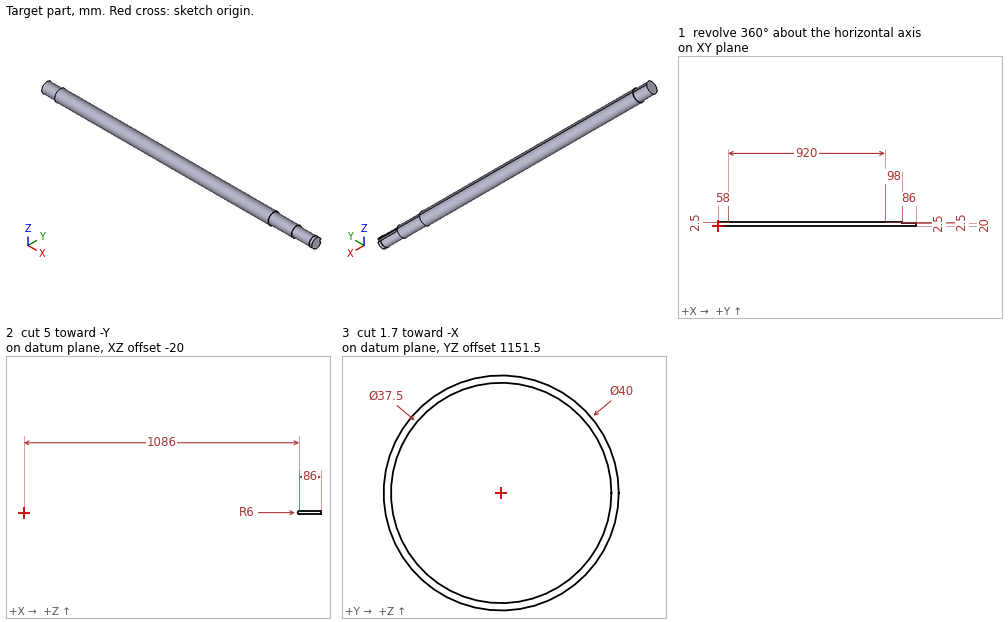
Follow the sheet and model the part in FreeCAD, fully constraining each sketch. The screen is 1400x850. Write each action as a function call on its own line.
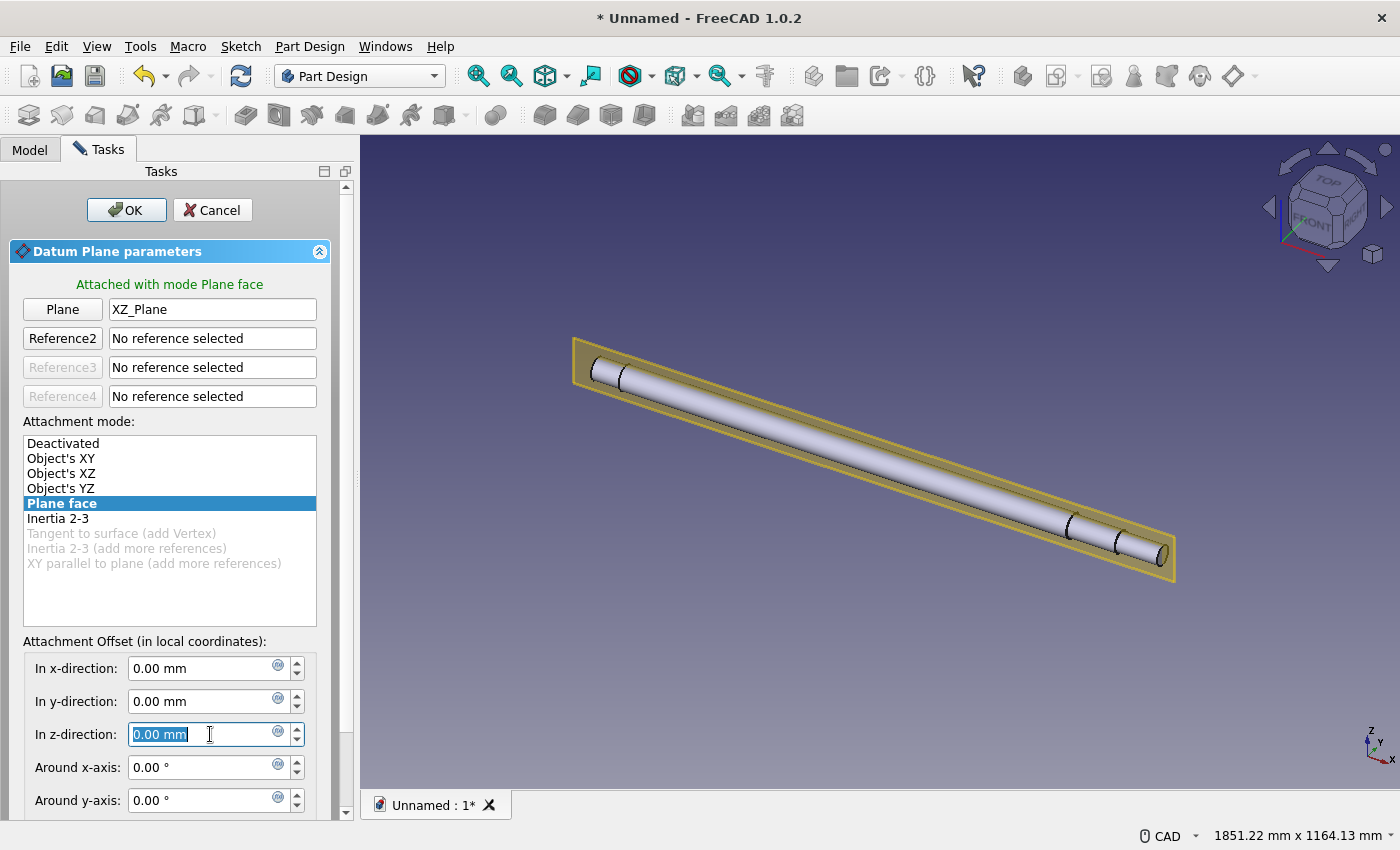
text(-20)
key(Tab)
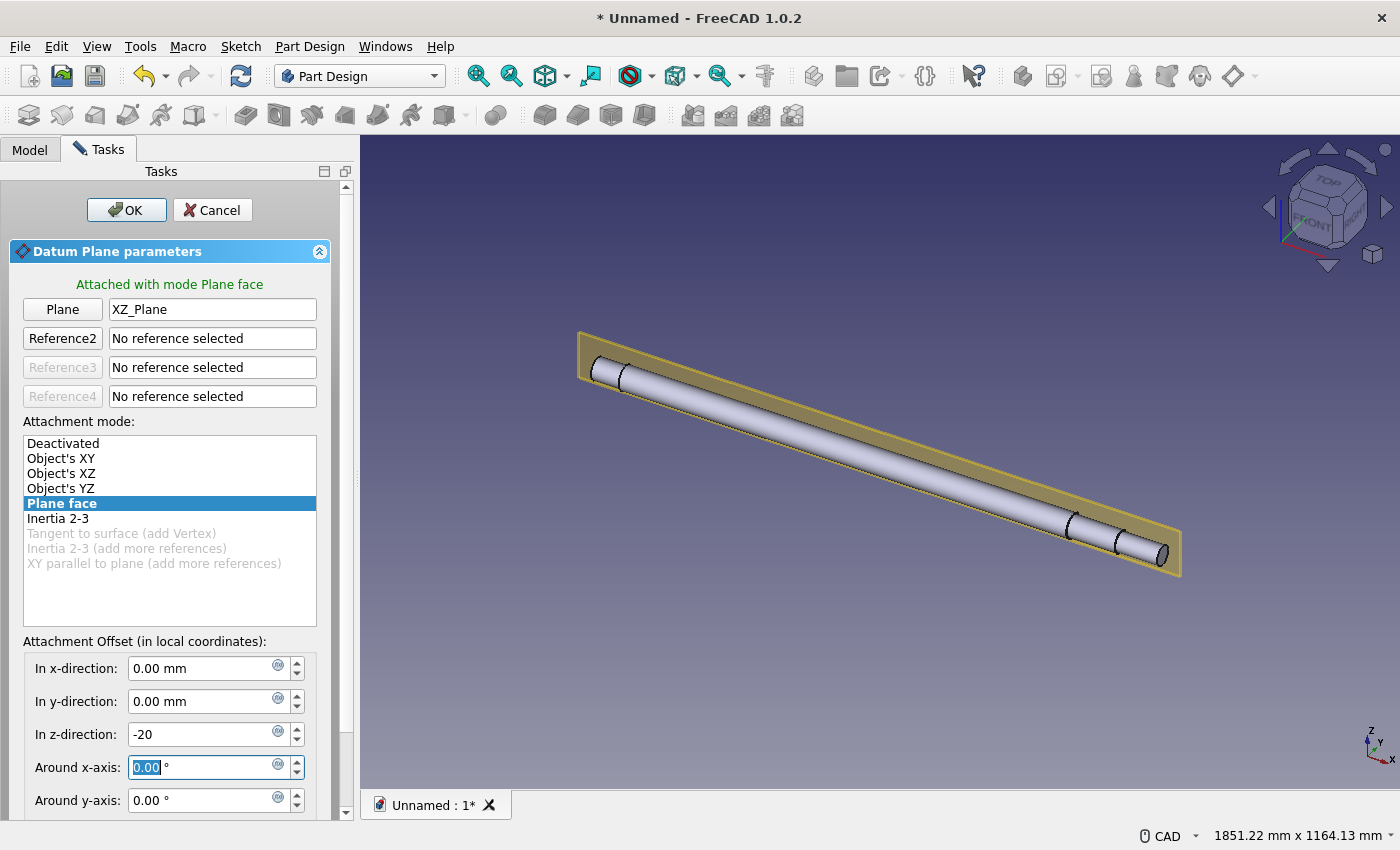
click(127, 210)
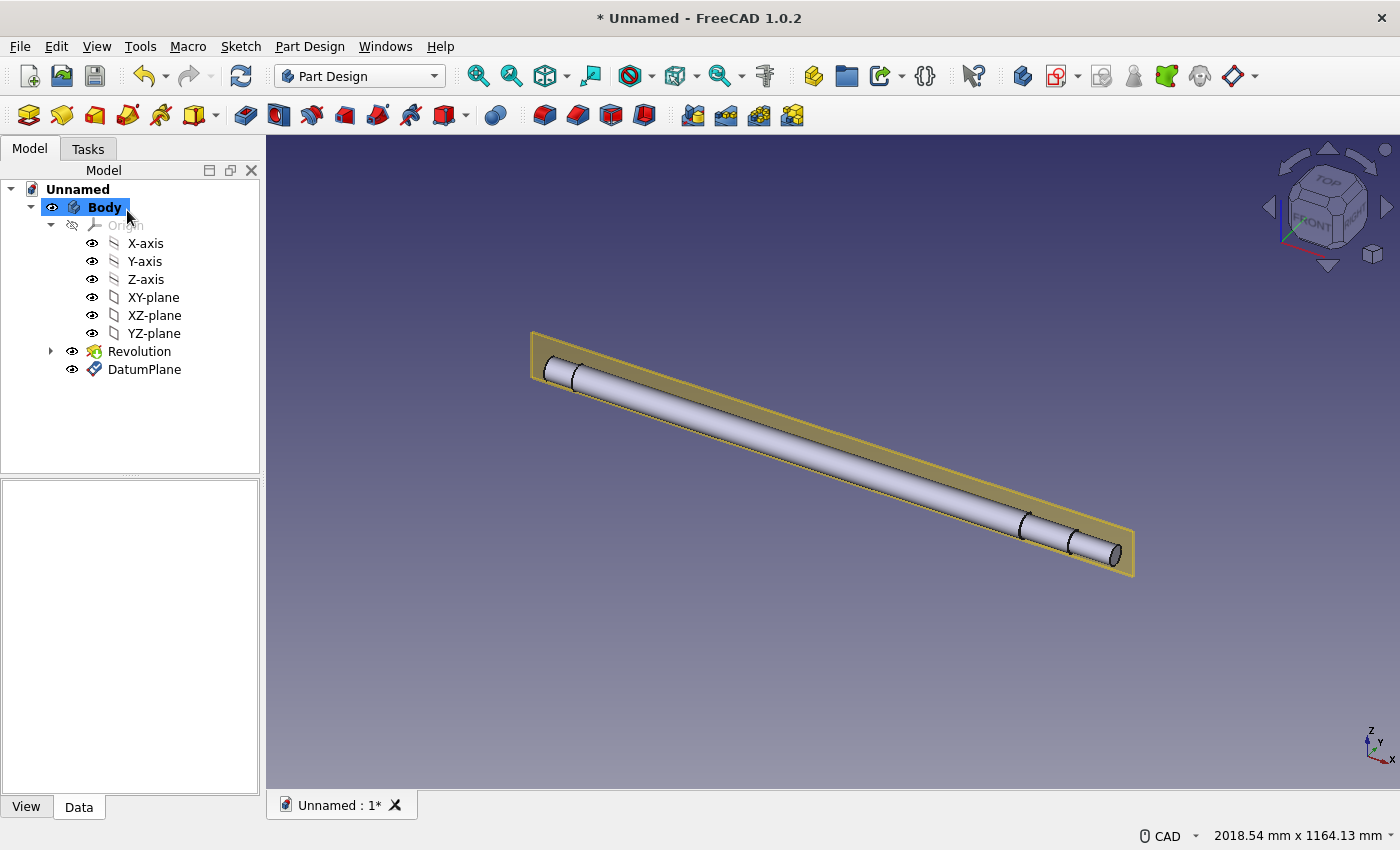
click(117, 369)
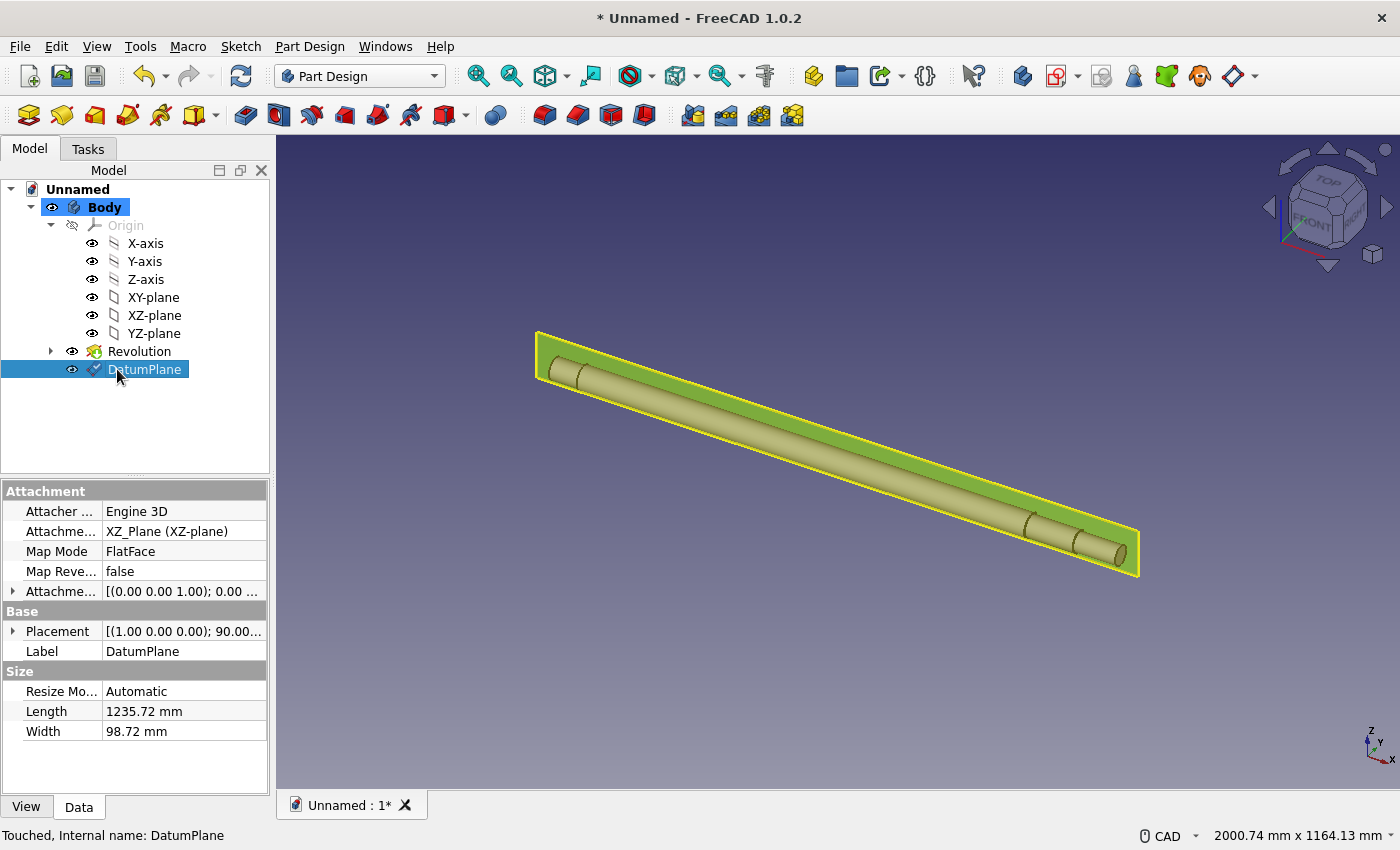
click(1056, 76)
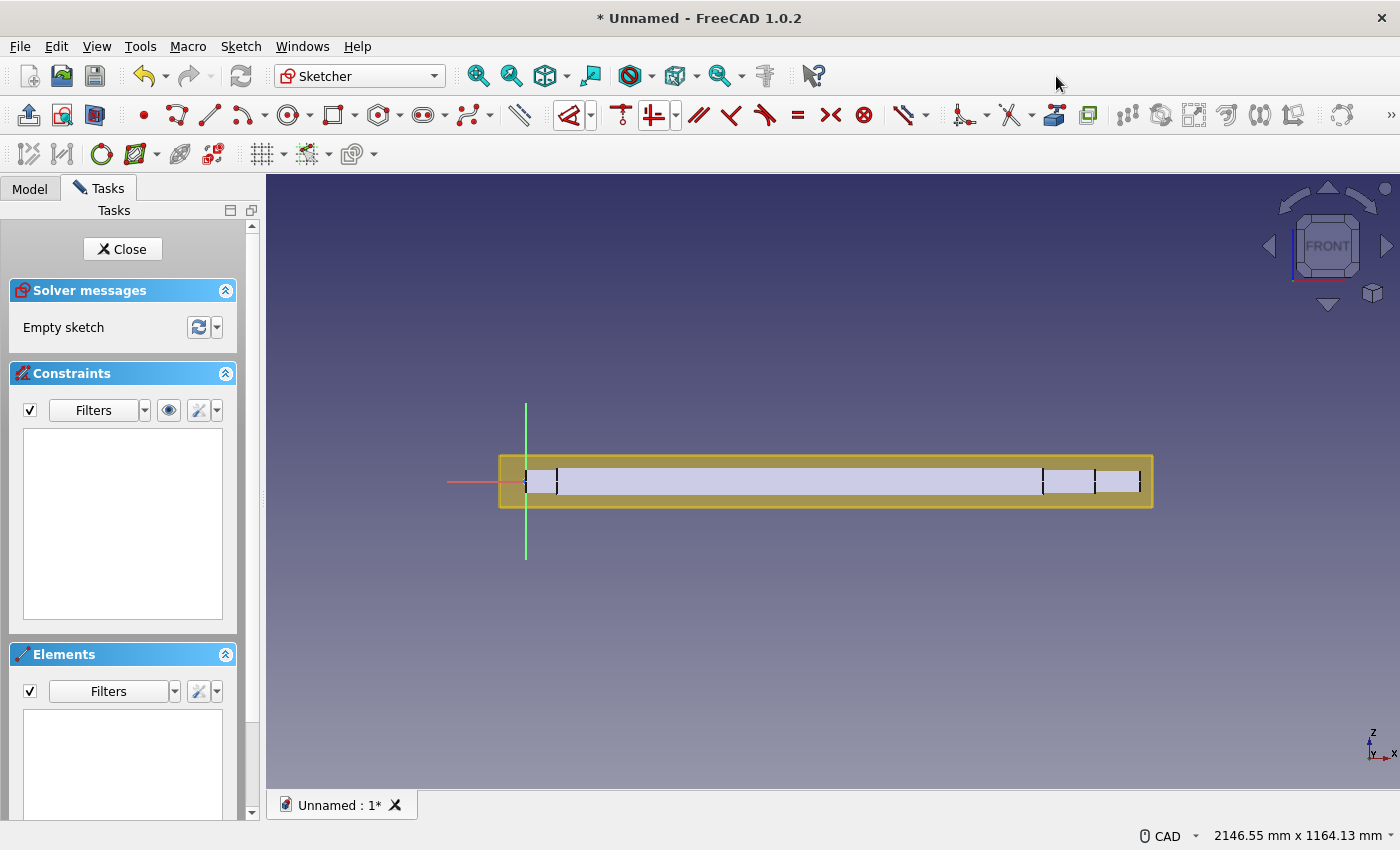
click(95, 116)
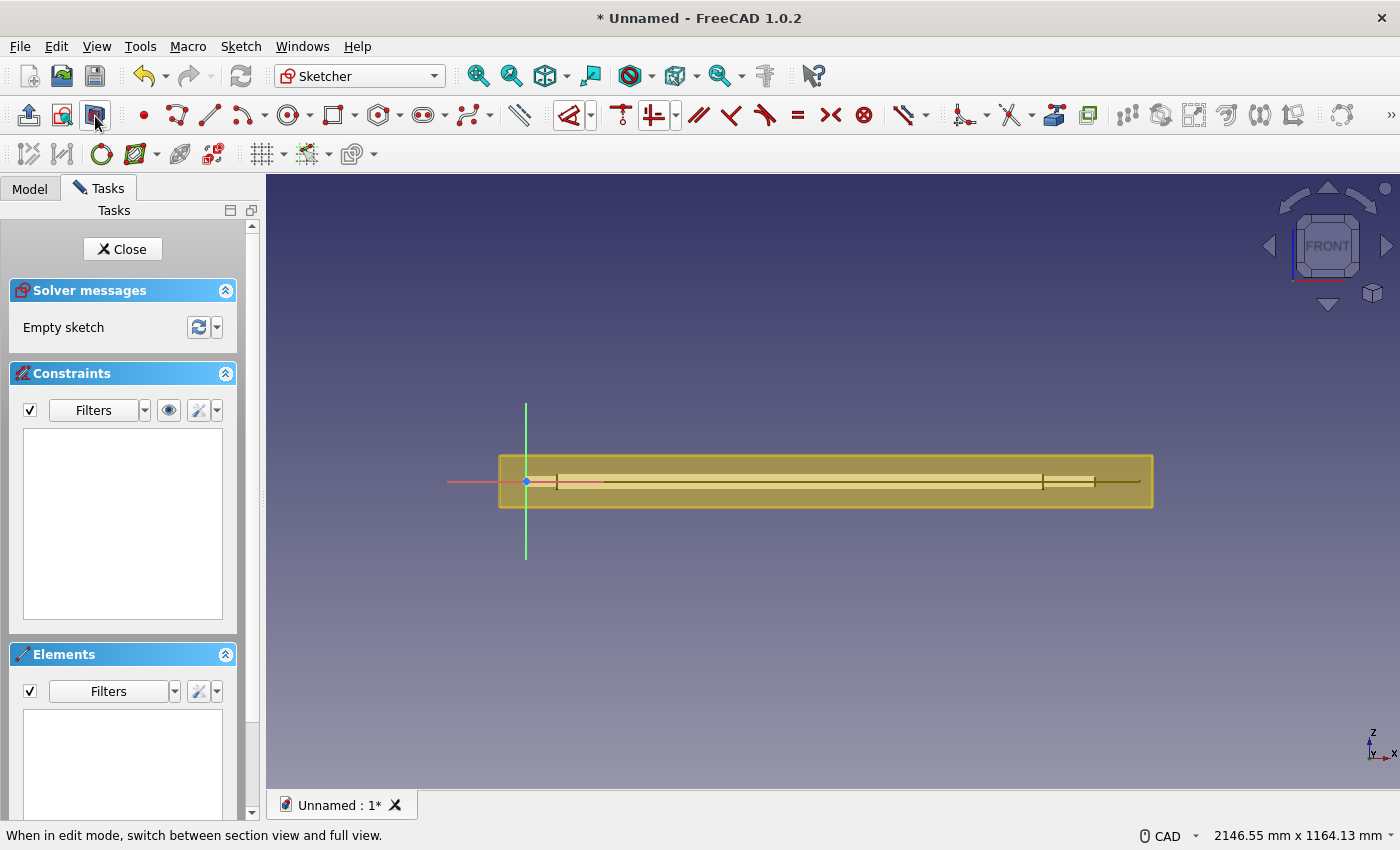
scroll(1150, 482, up, 13)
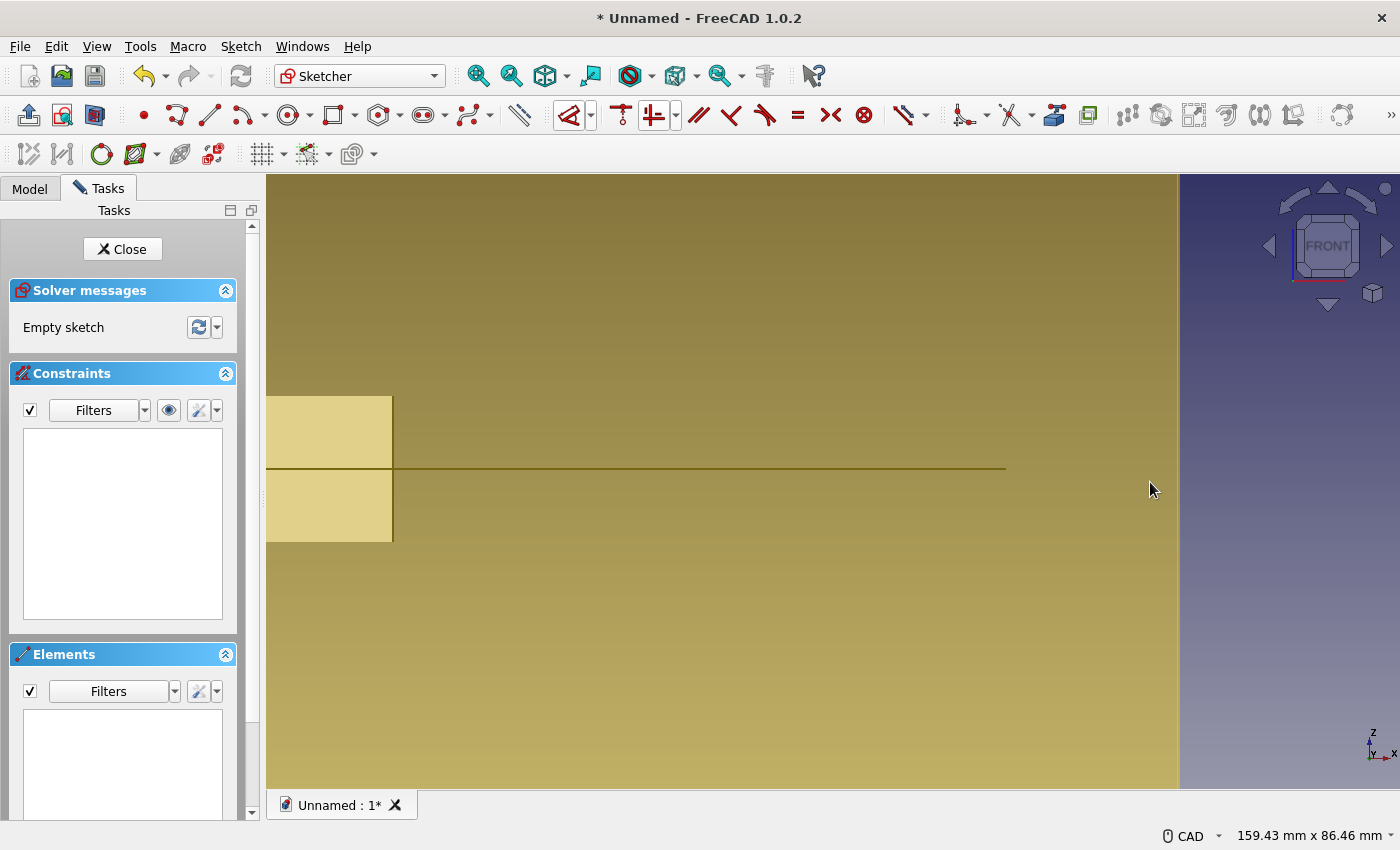
click(177, 116)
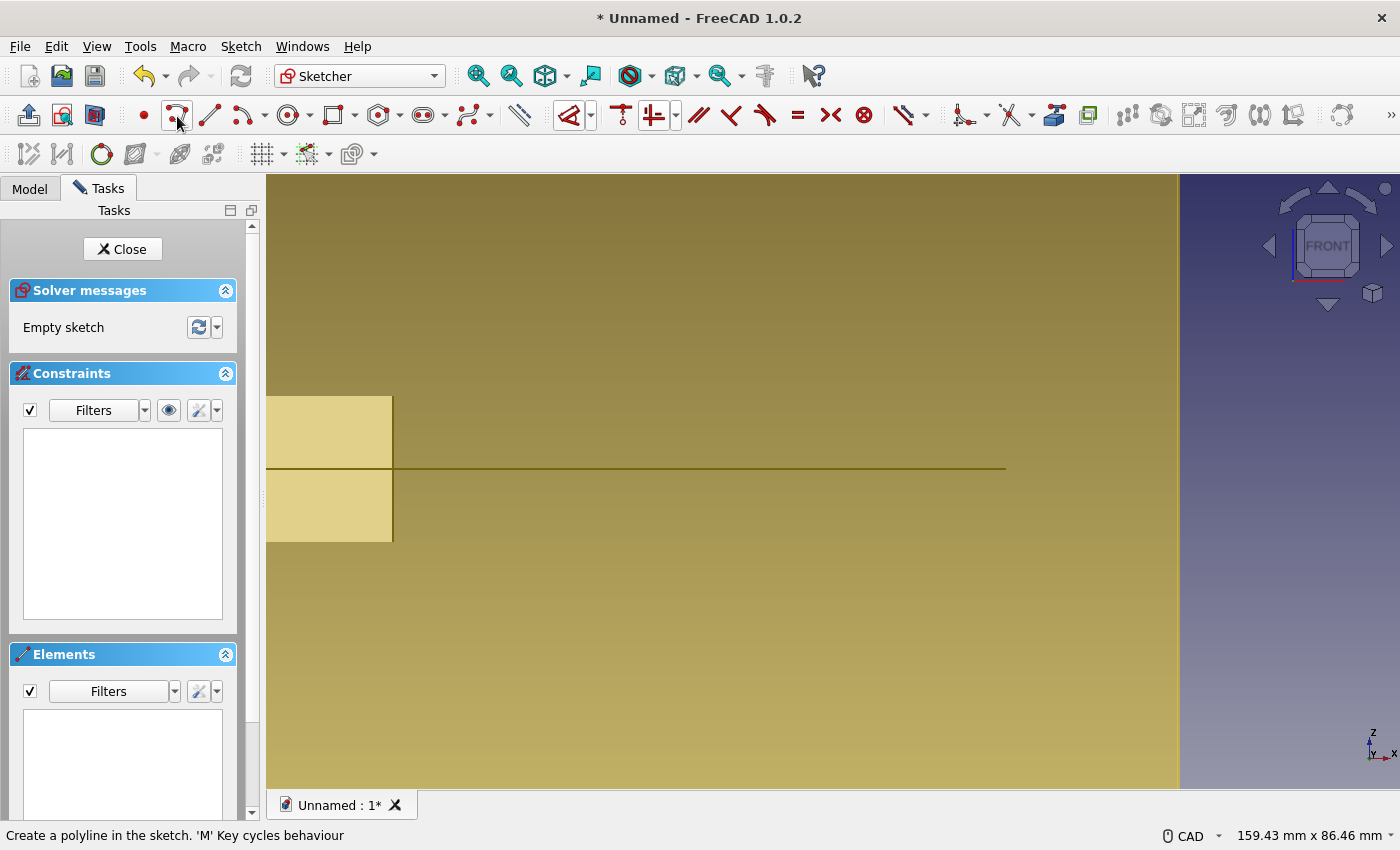
click(464, 426)
click(1076, 426)
click(1076, 512)
click(464, 512)
right_click(464, 512)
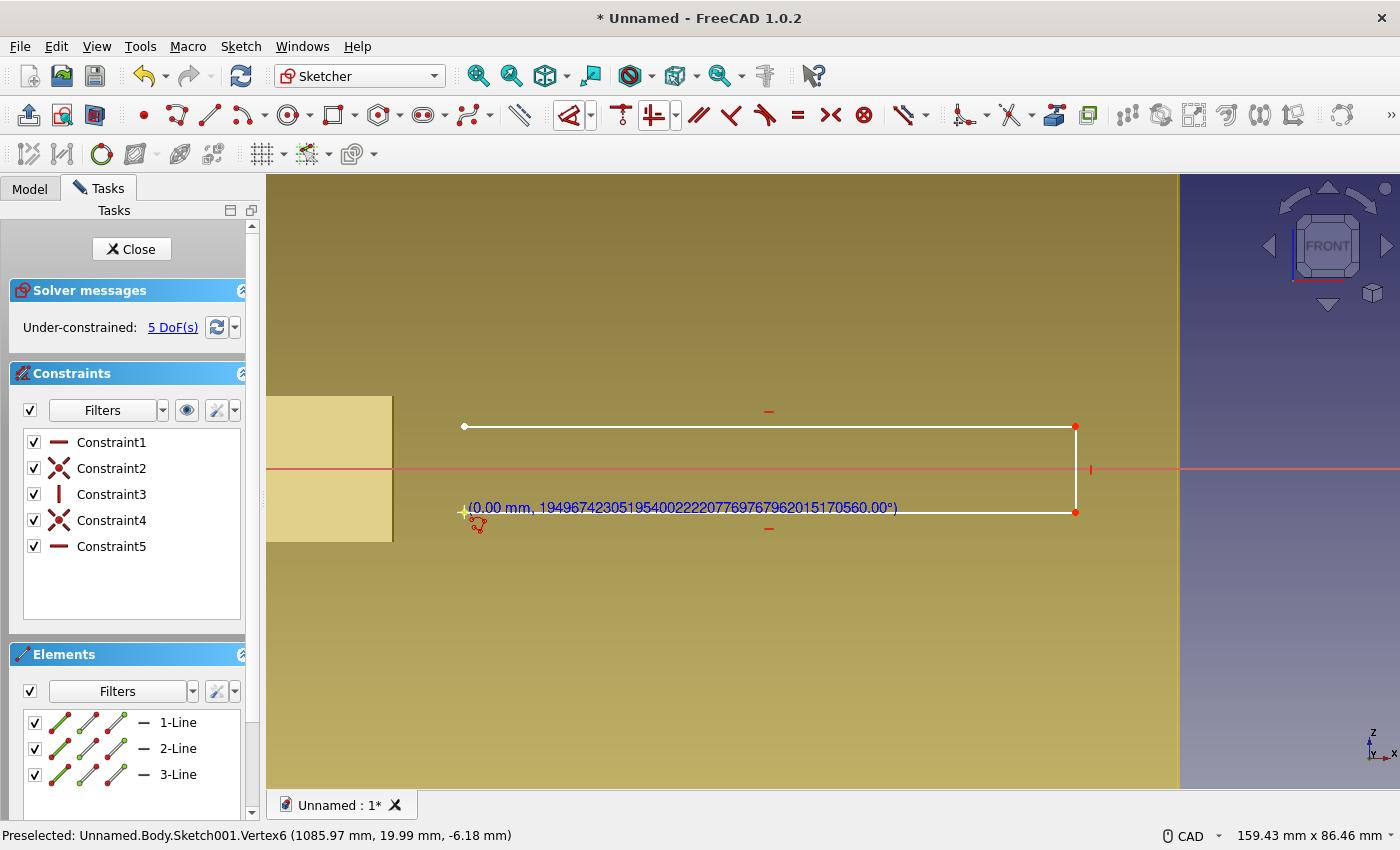
key(g)
key(3)
key(a)